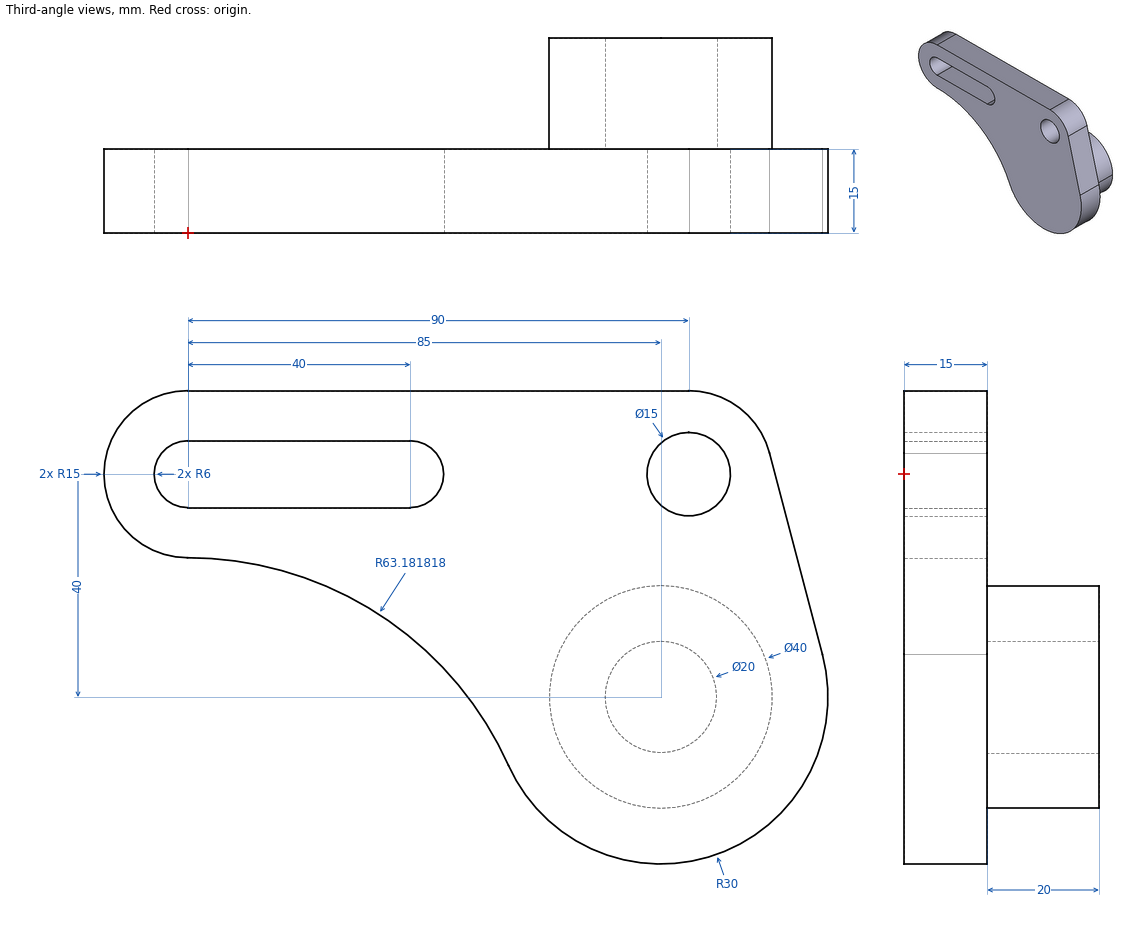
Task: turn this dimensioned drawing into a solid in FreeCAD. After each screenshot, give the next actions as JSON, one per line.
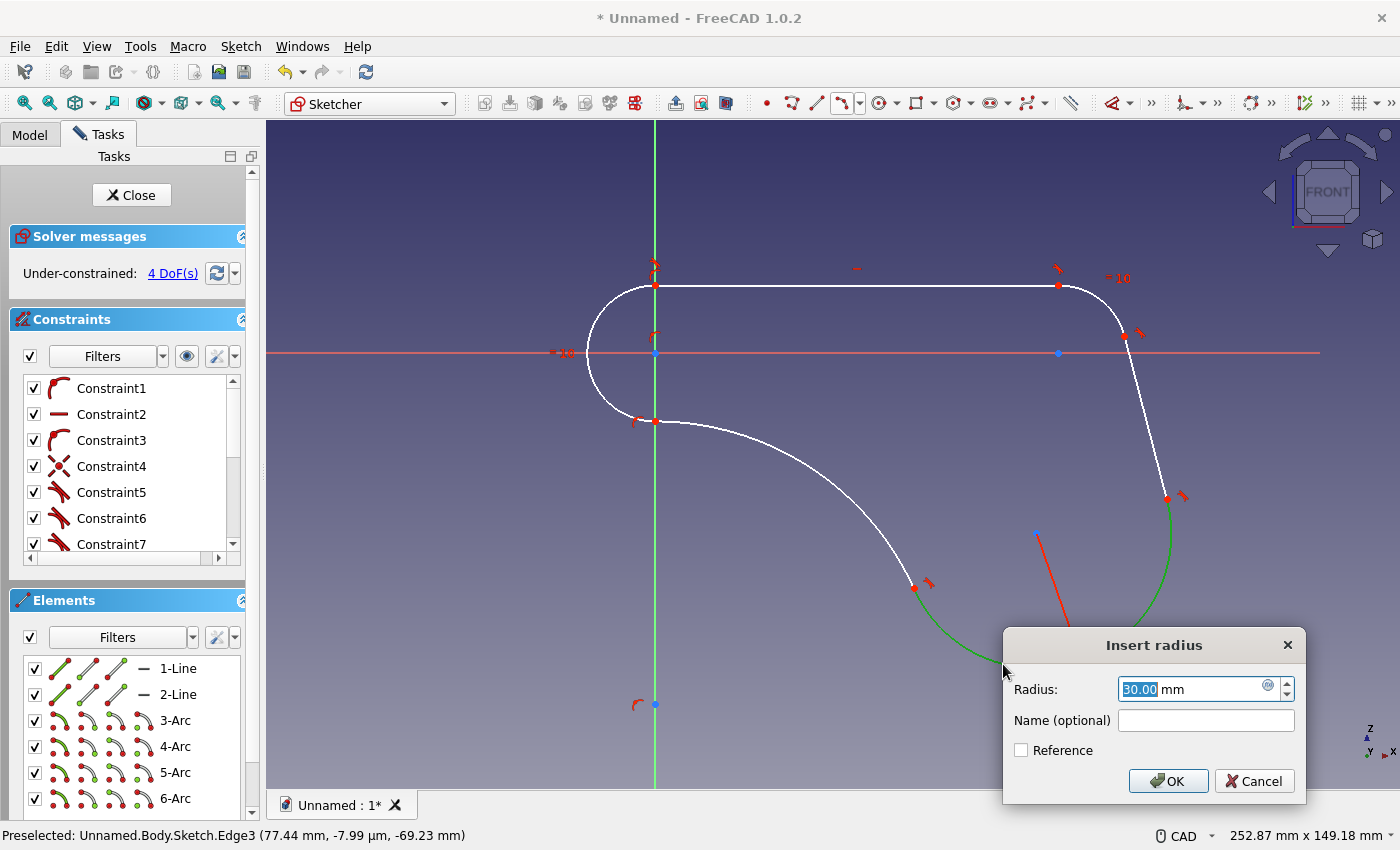
{"action": "type", "text": "30"}
{"action": "key", "text": "Return"}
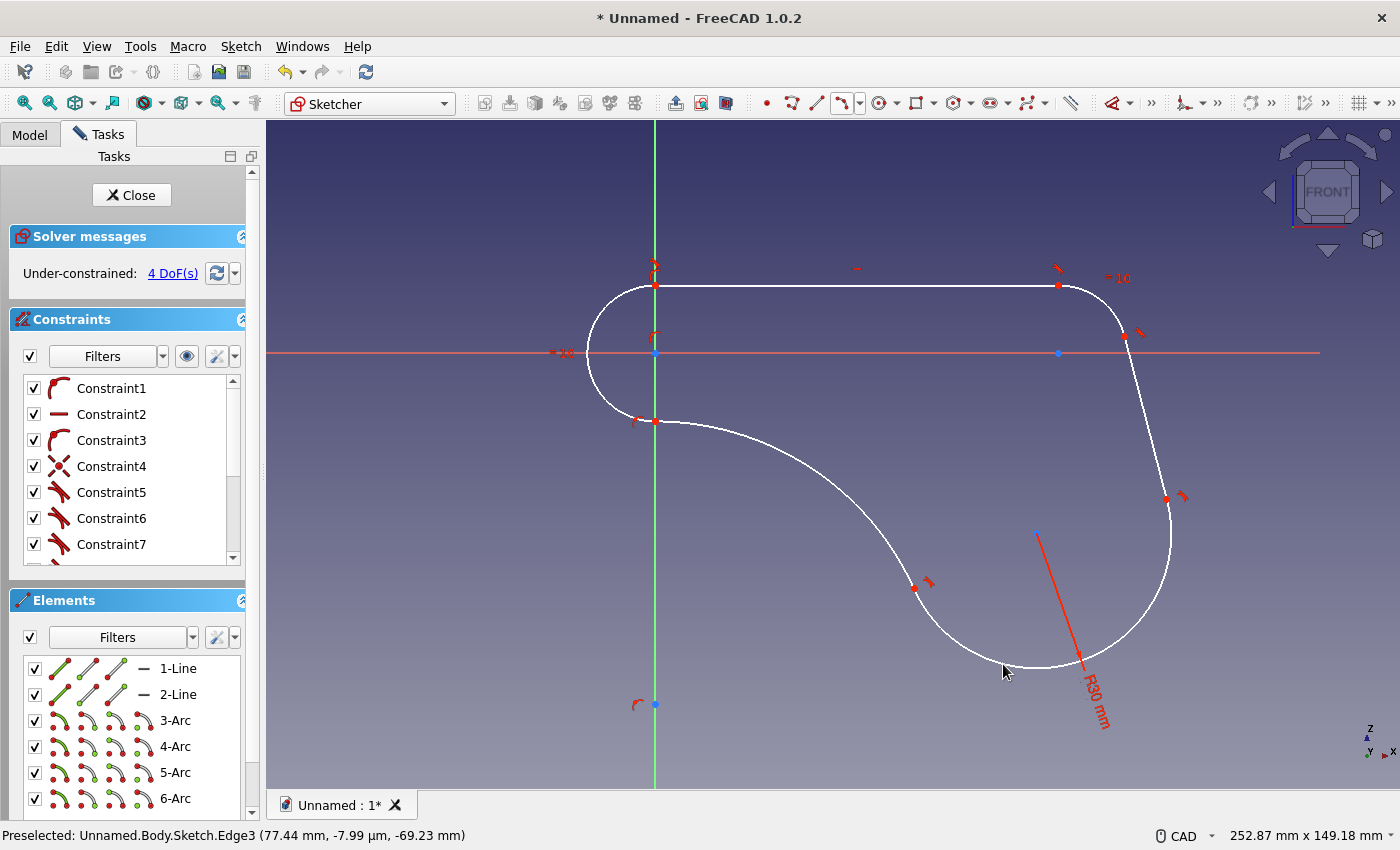
{"action": "left_click", "coordinate": [860, 508]}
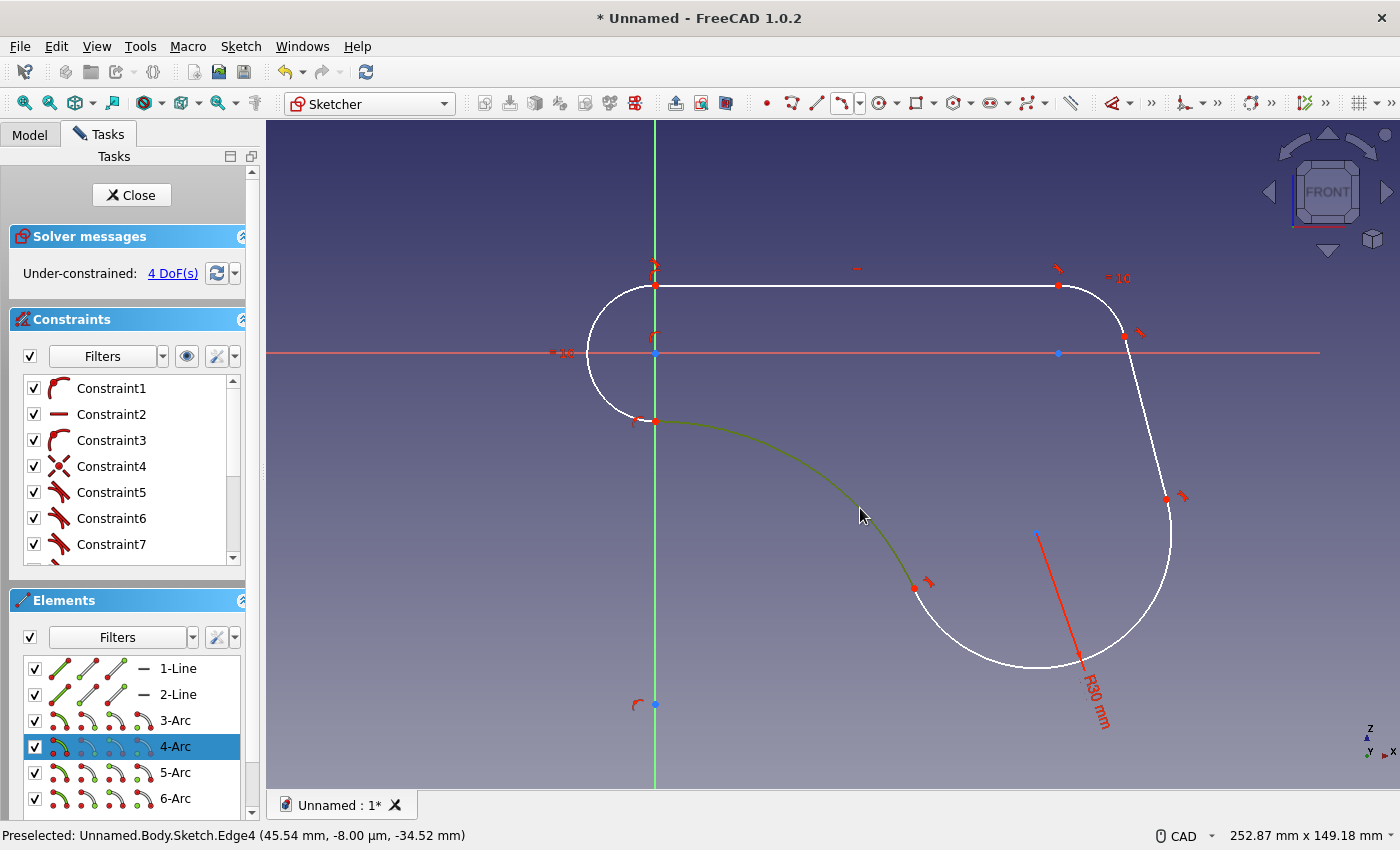
{"action": "left_click", "coordinate": [1130, 104]}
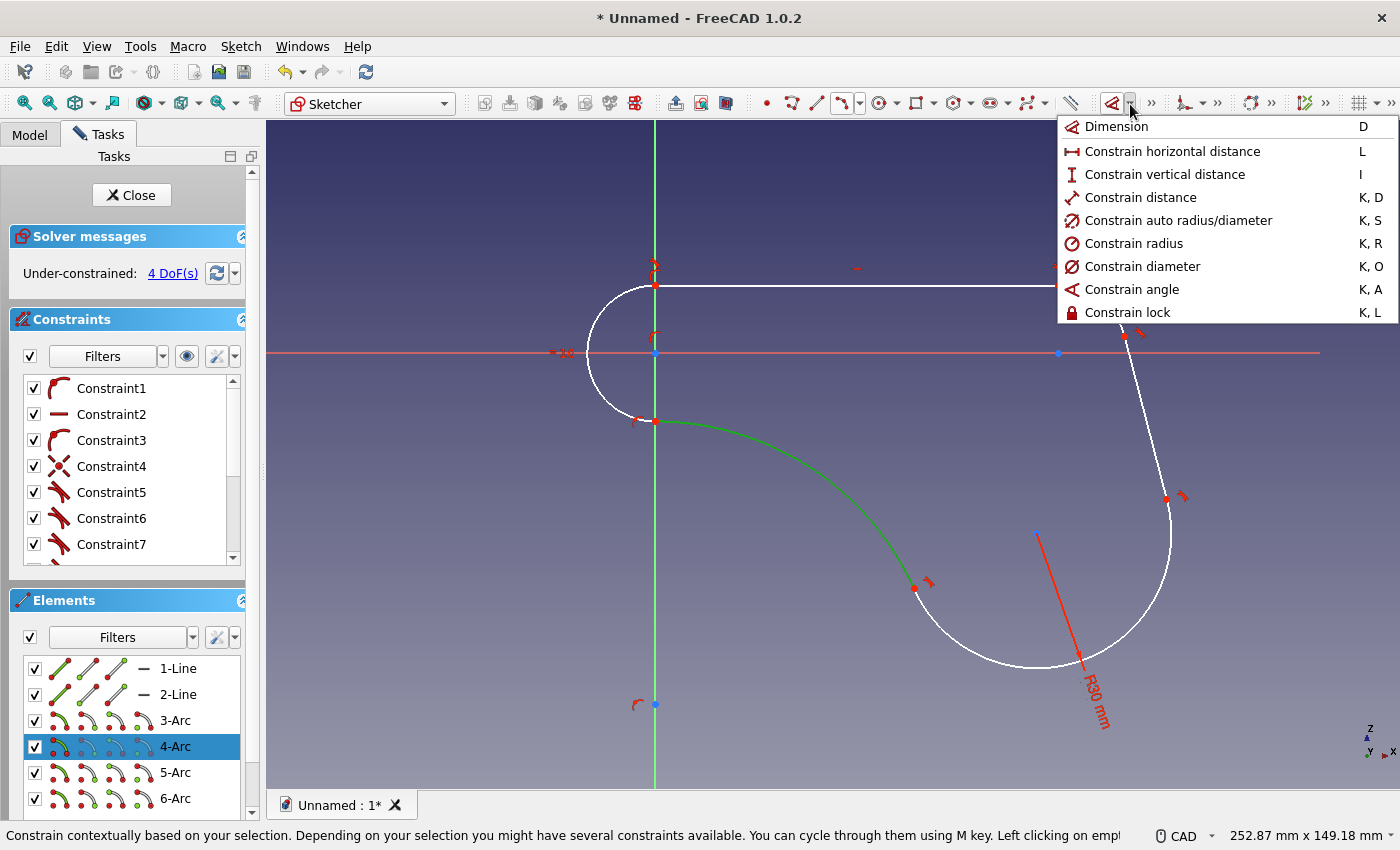
{"action": "left_click", "coordinate": [1228, 244]}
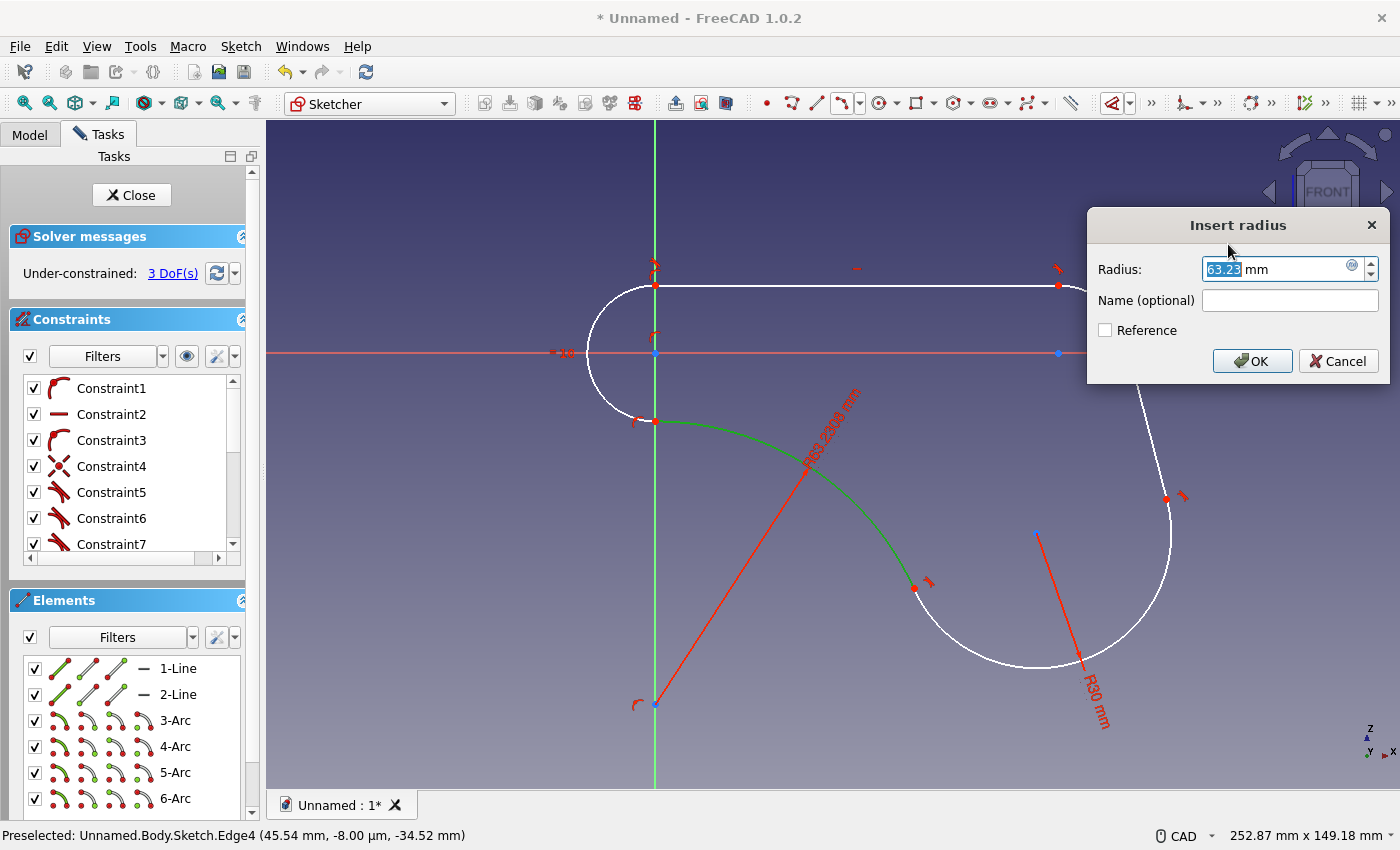
{"action": "type", "text": "63.181818"}
{"action": "key", "text": "Return"}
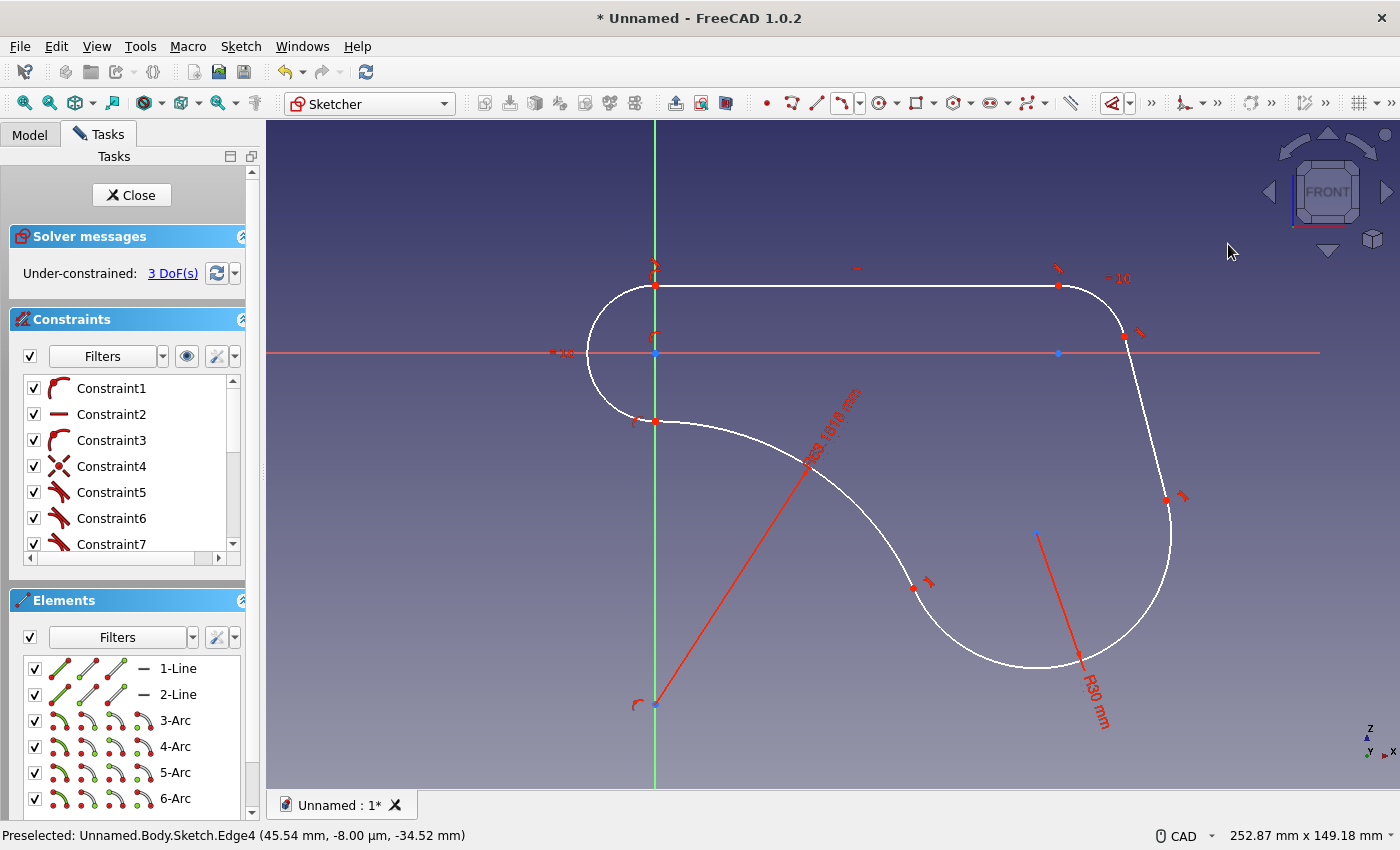
{"action": "left_click", "coordinate": [600, 314]}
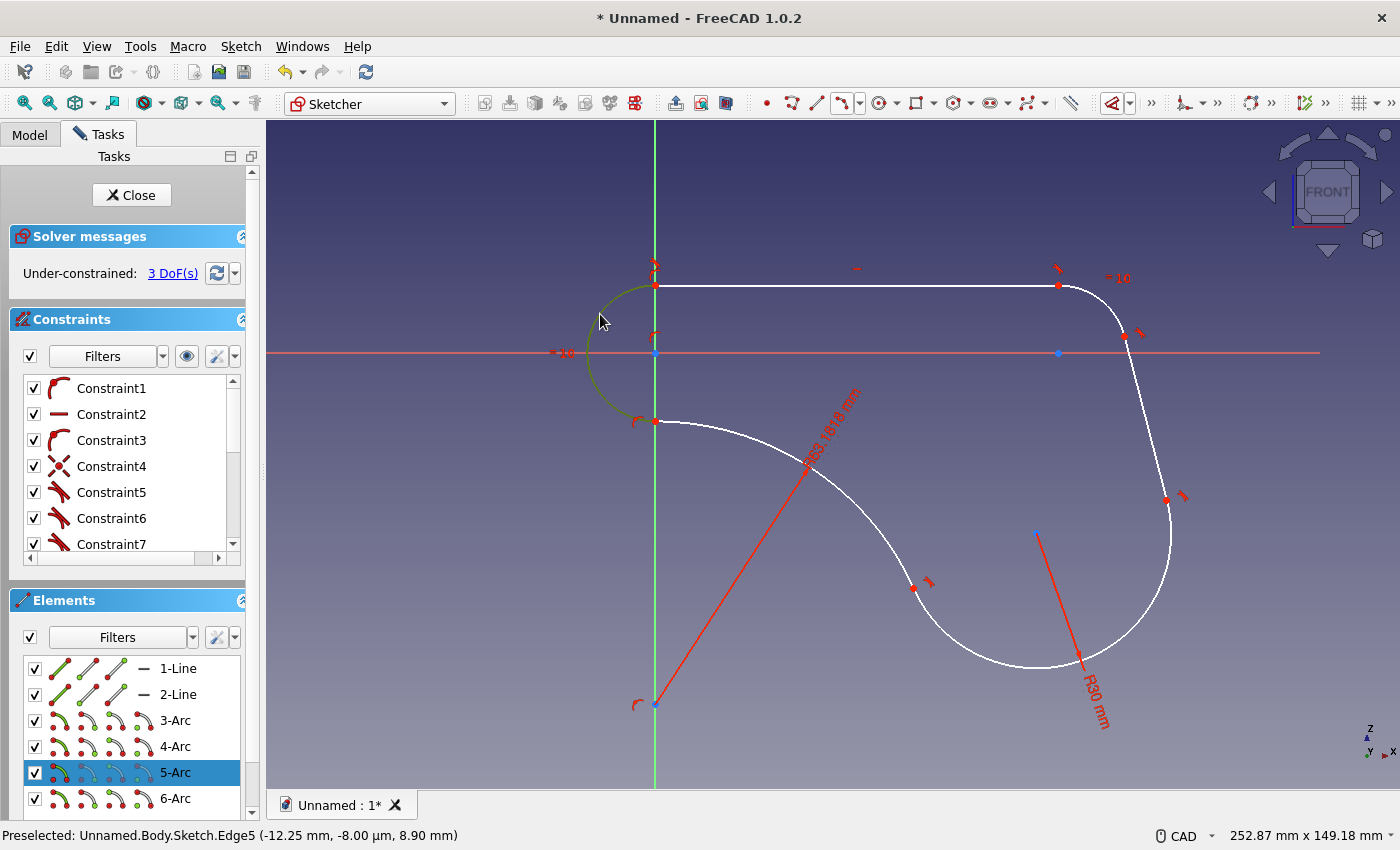
{"action": "left_click", "coordinate": [1130, 104]}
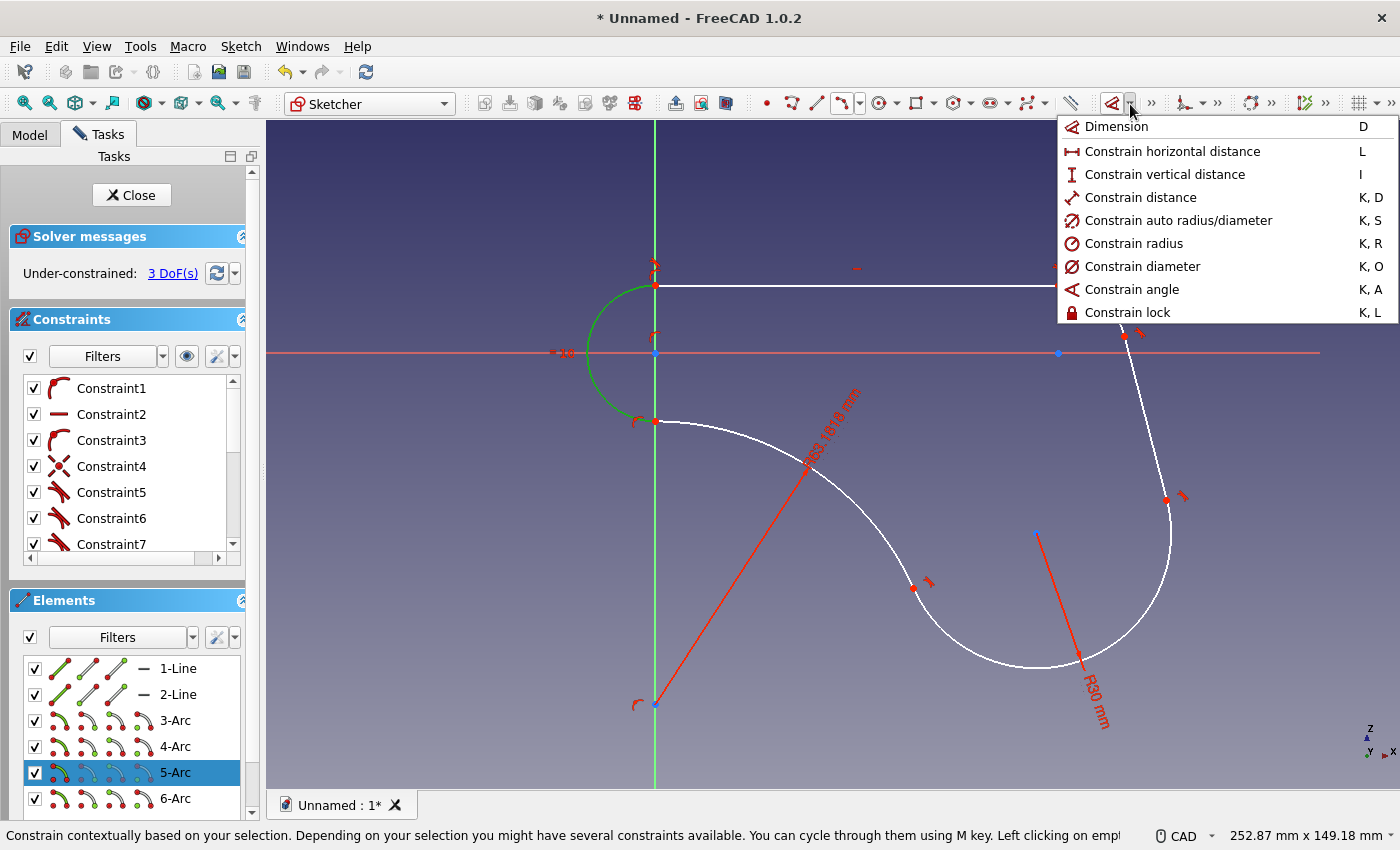
{"action": "left_click", "coordinate": [1228, 244]}